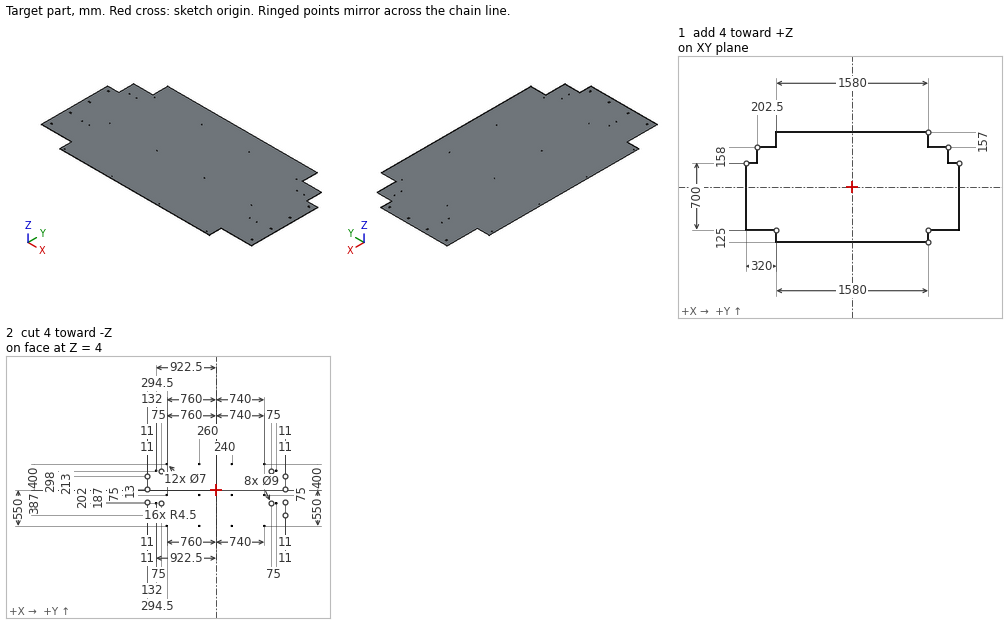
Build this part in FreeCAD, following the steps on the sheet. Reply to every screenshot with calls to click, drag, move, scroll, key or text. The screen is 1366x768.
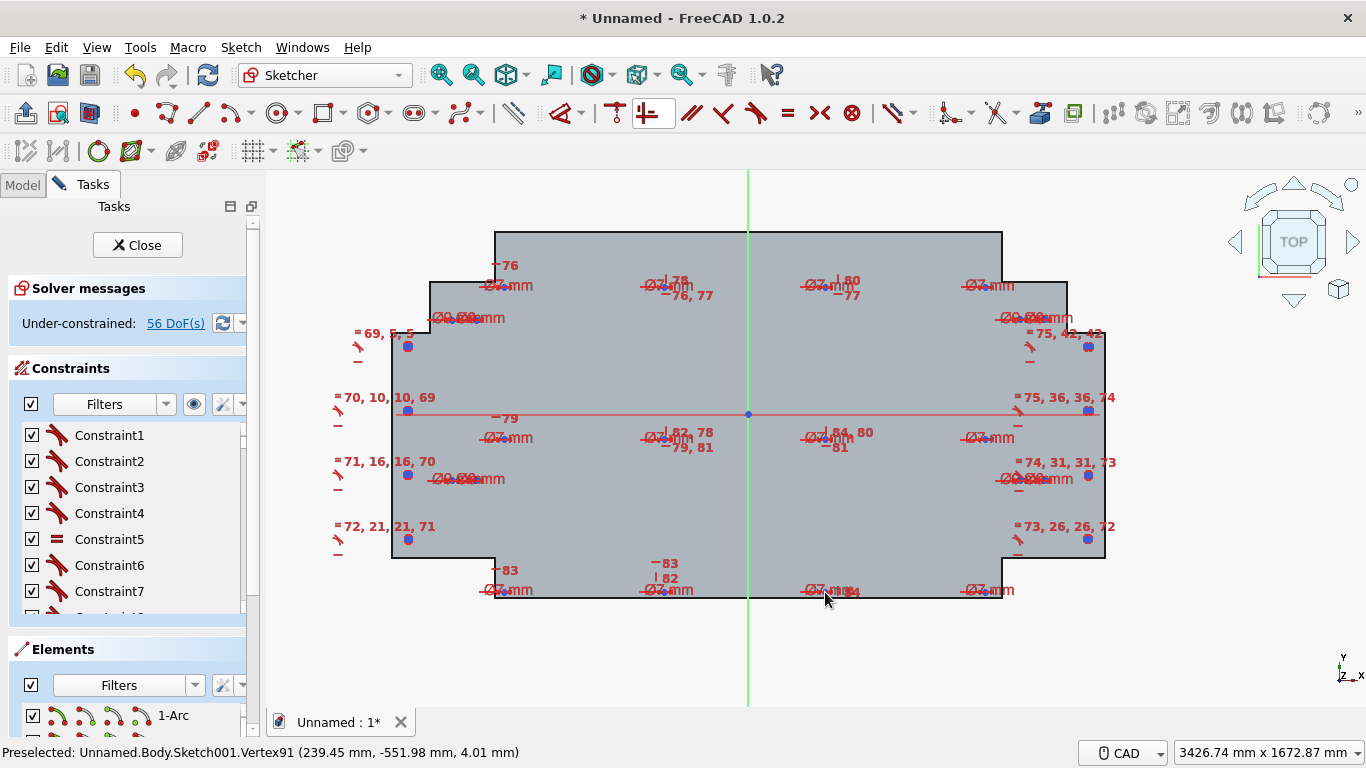
click(665, 592)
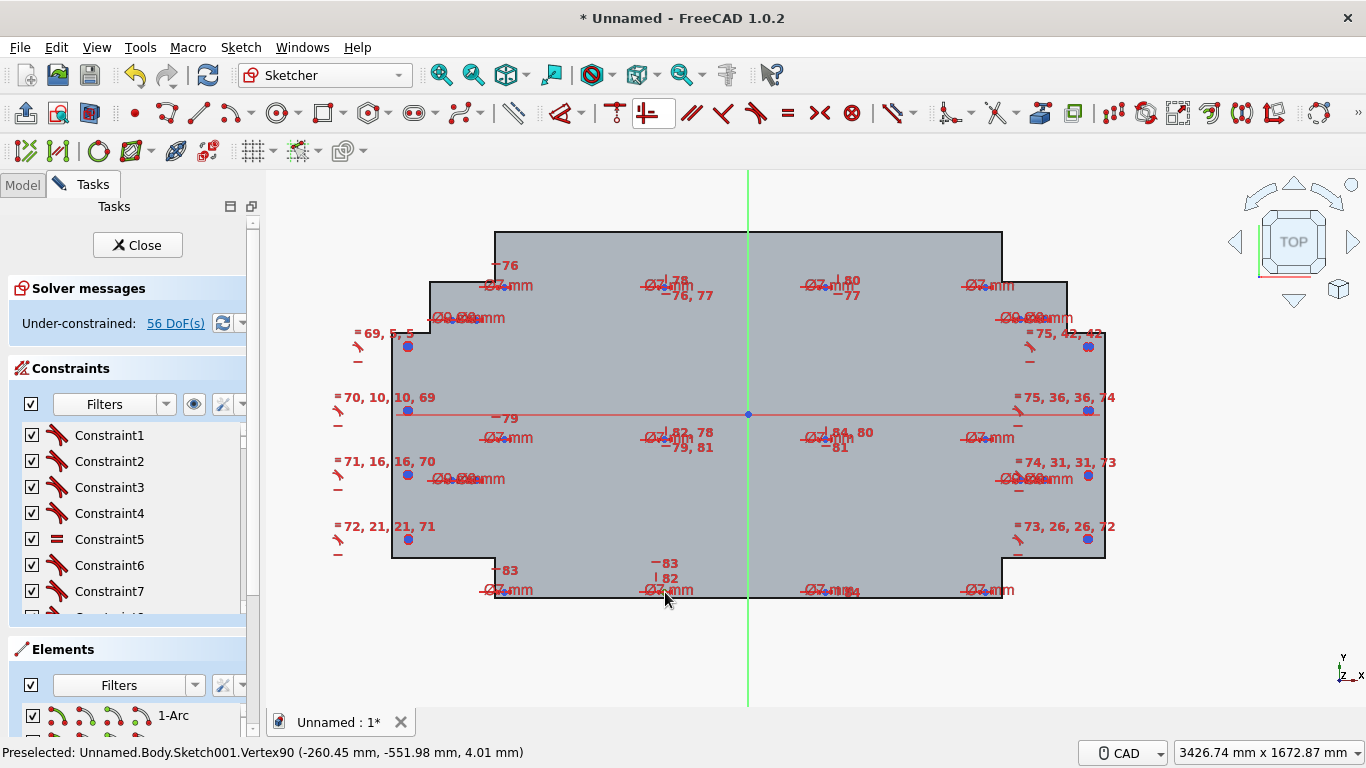
click(825, 592)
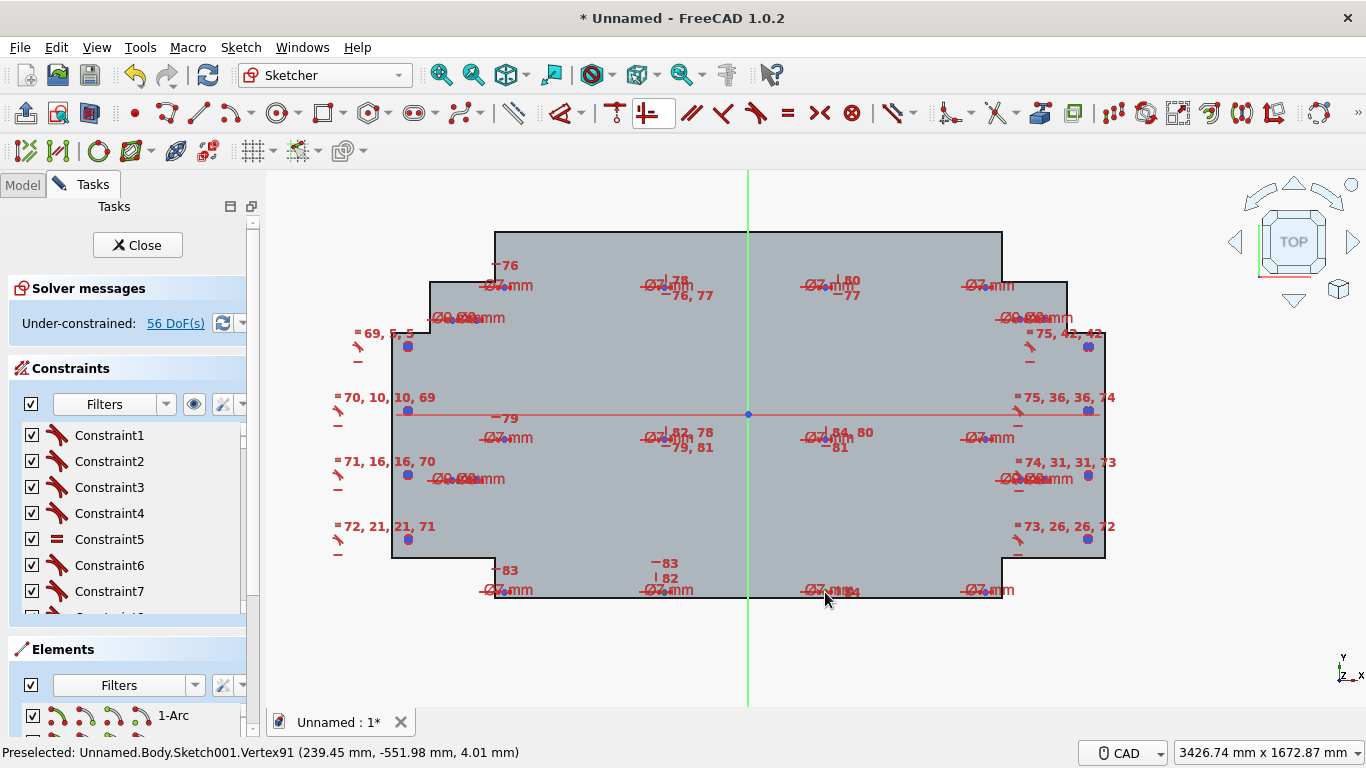
key(h)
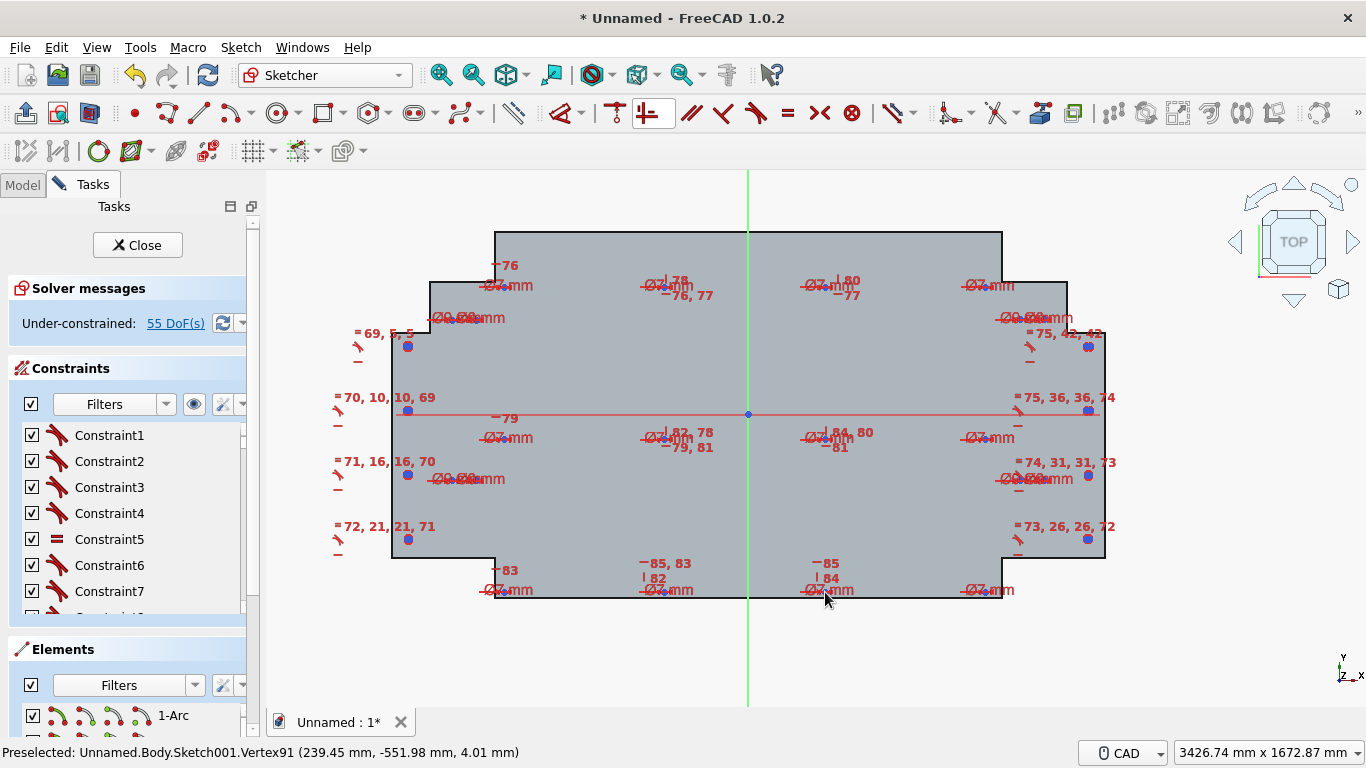
click(452, 320)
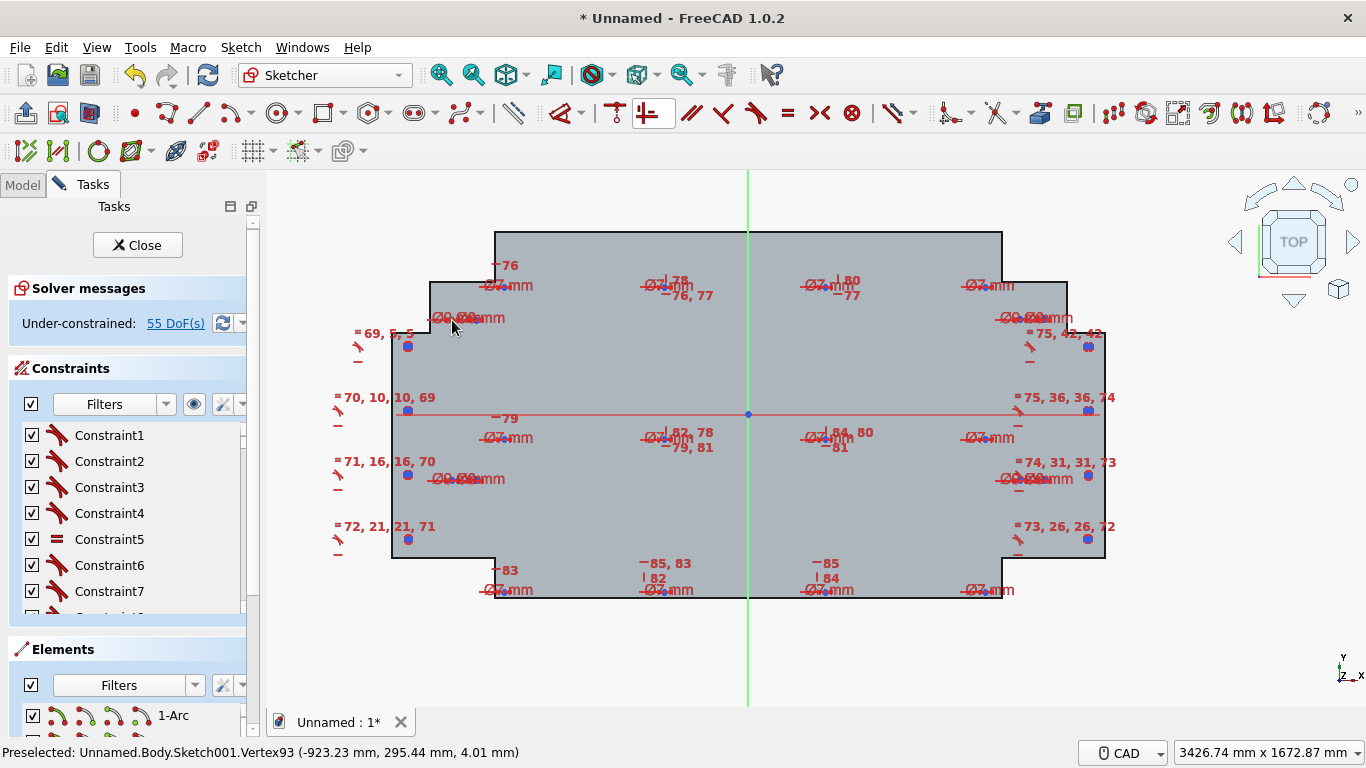
click(476, 320)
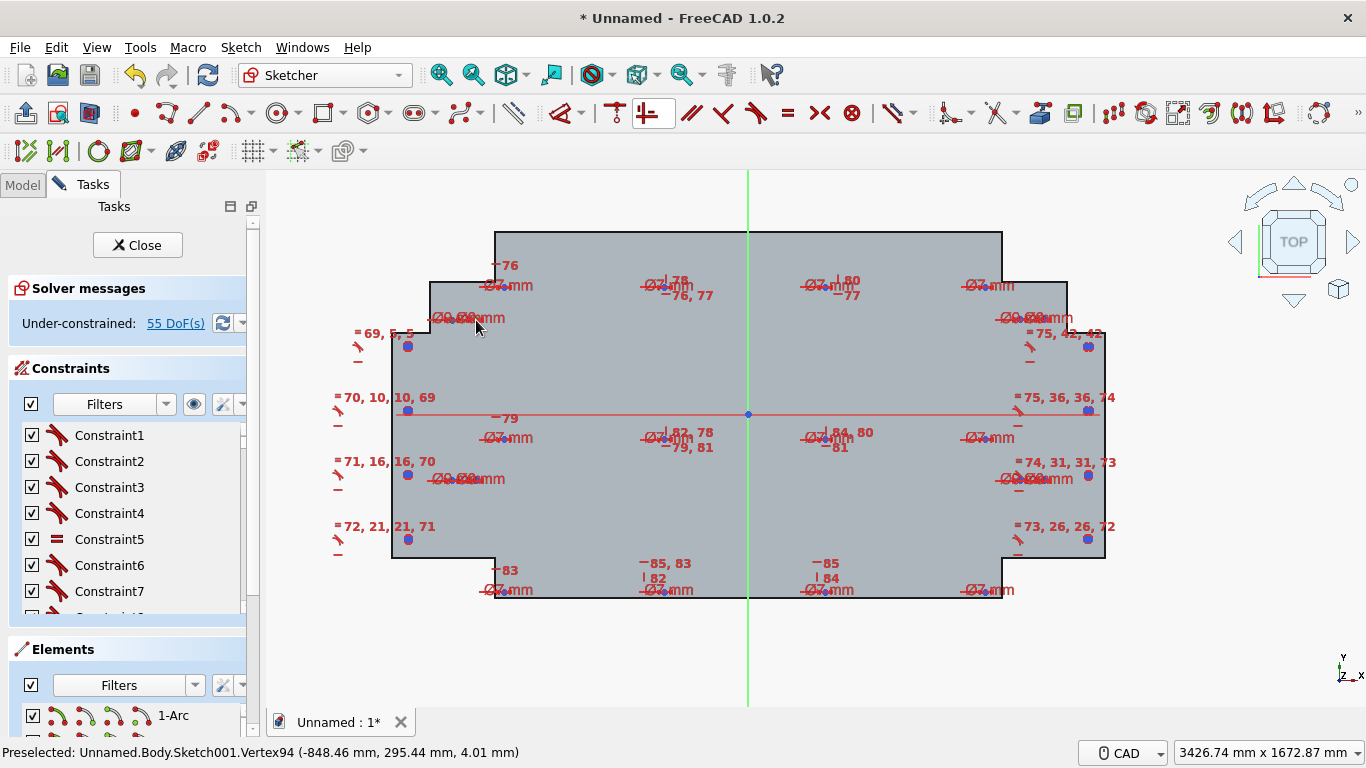
key(h)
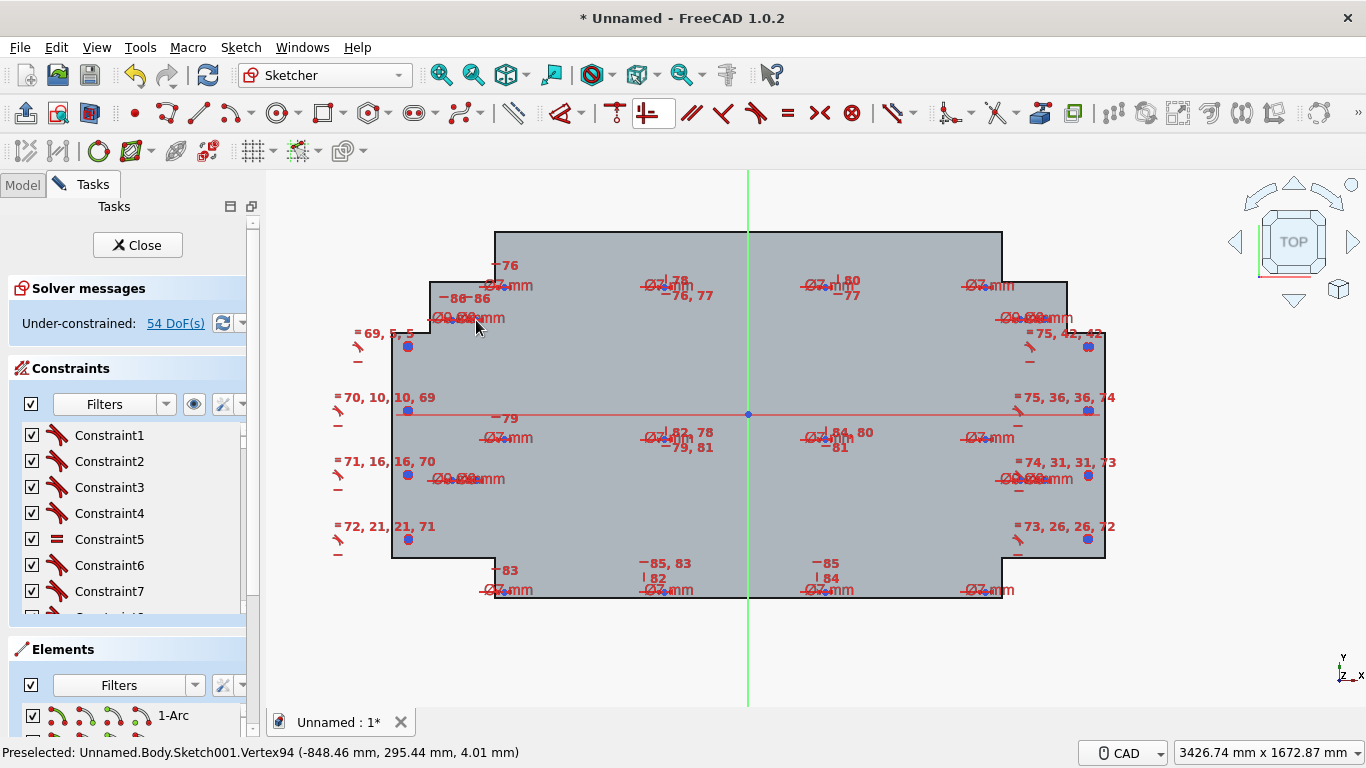
click(452, 481)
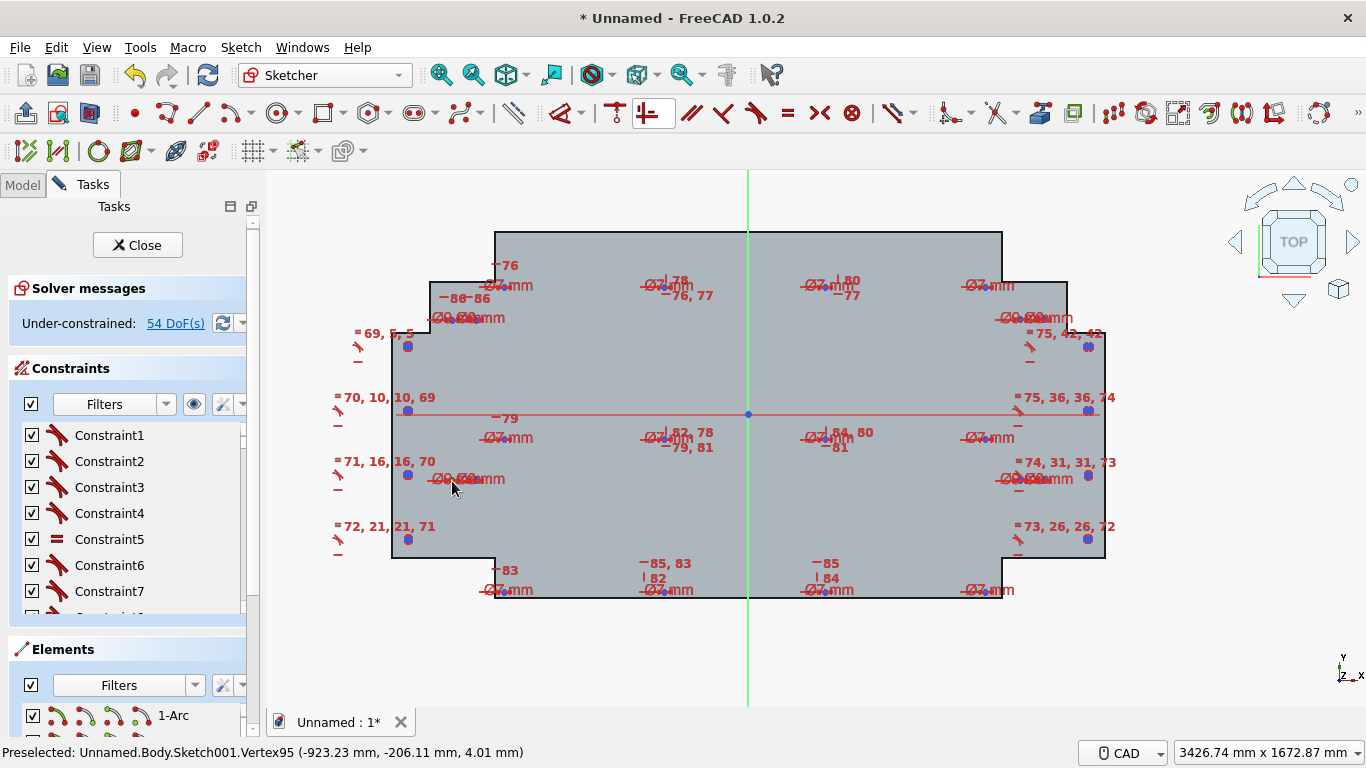
click(476, 481)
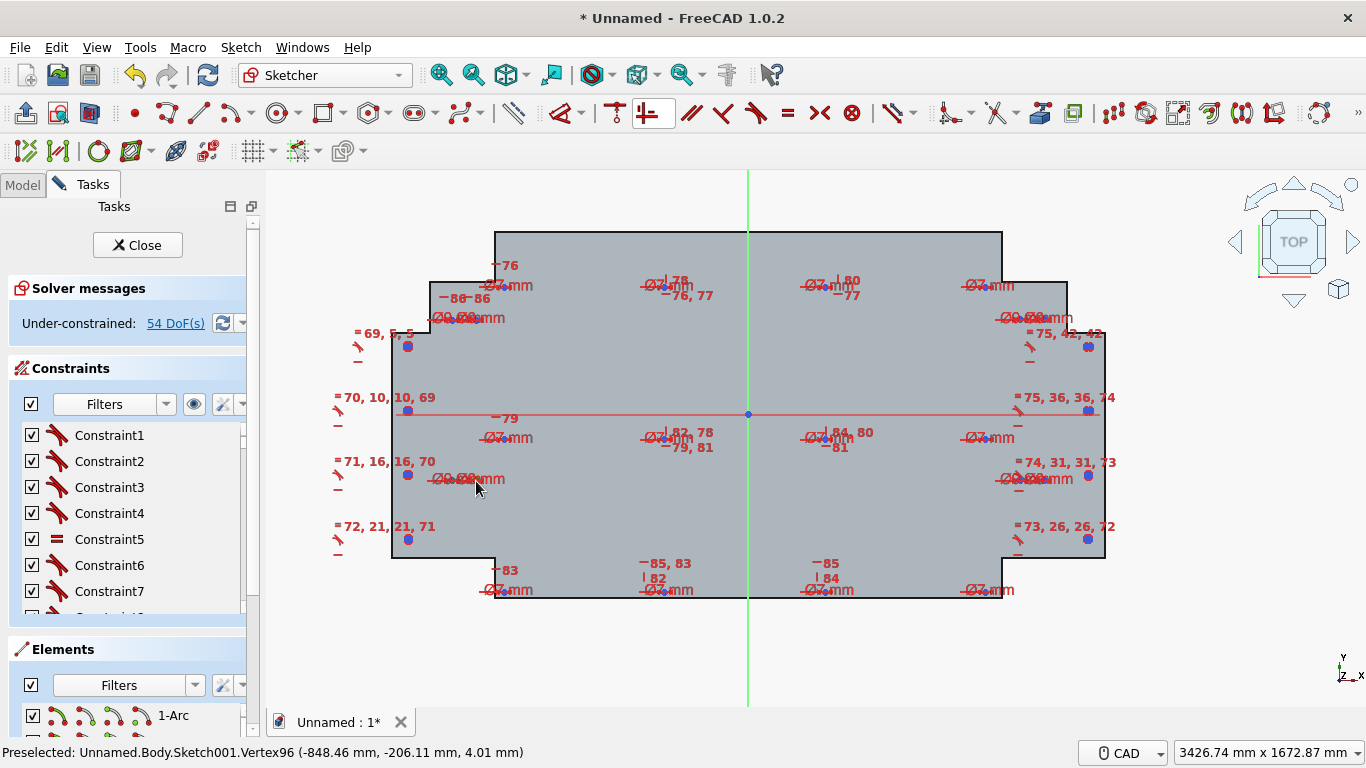
key(h)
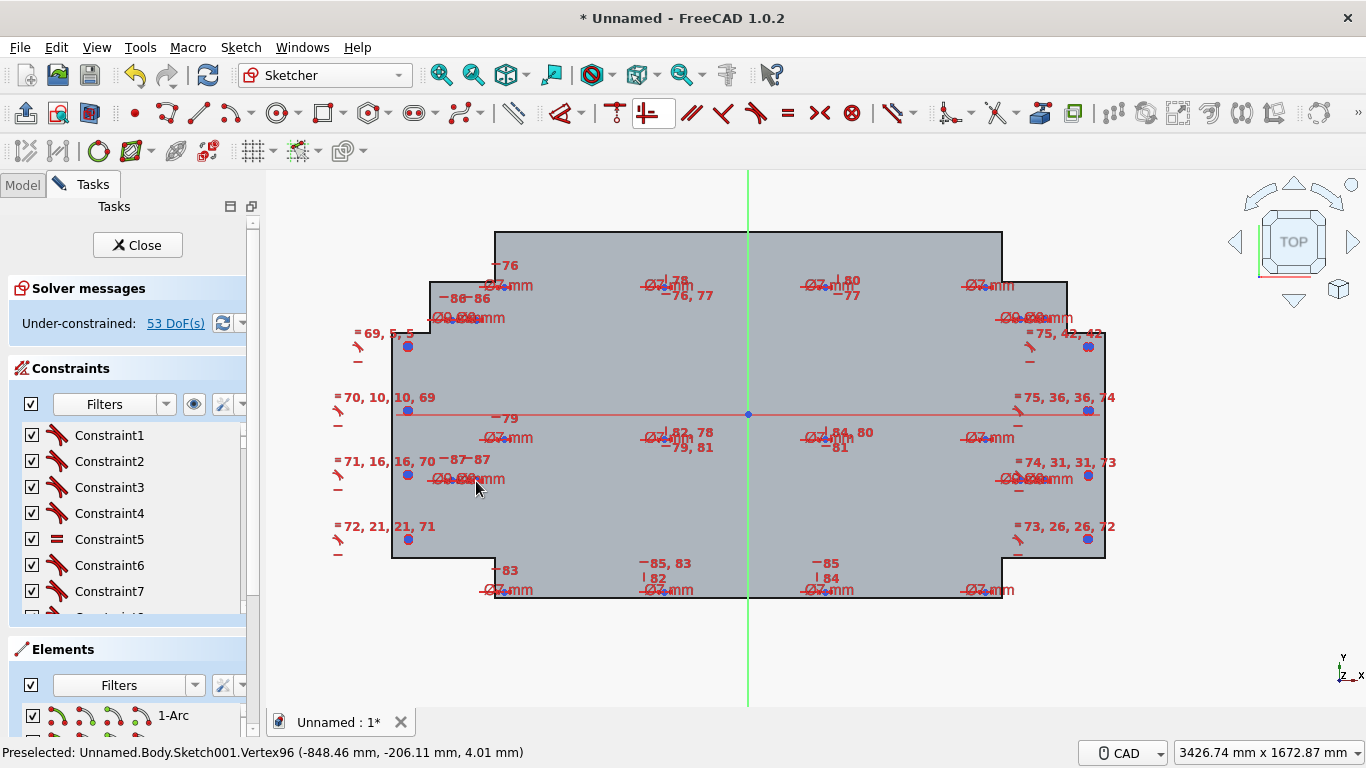
click(1020, 320)